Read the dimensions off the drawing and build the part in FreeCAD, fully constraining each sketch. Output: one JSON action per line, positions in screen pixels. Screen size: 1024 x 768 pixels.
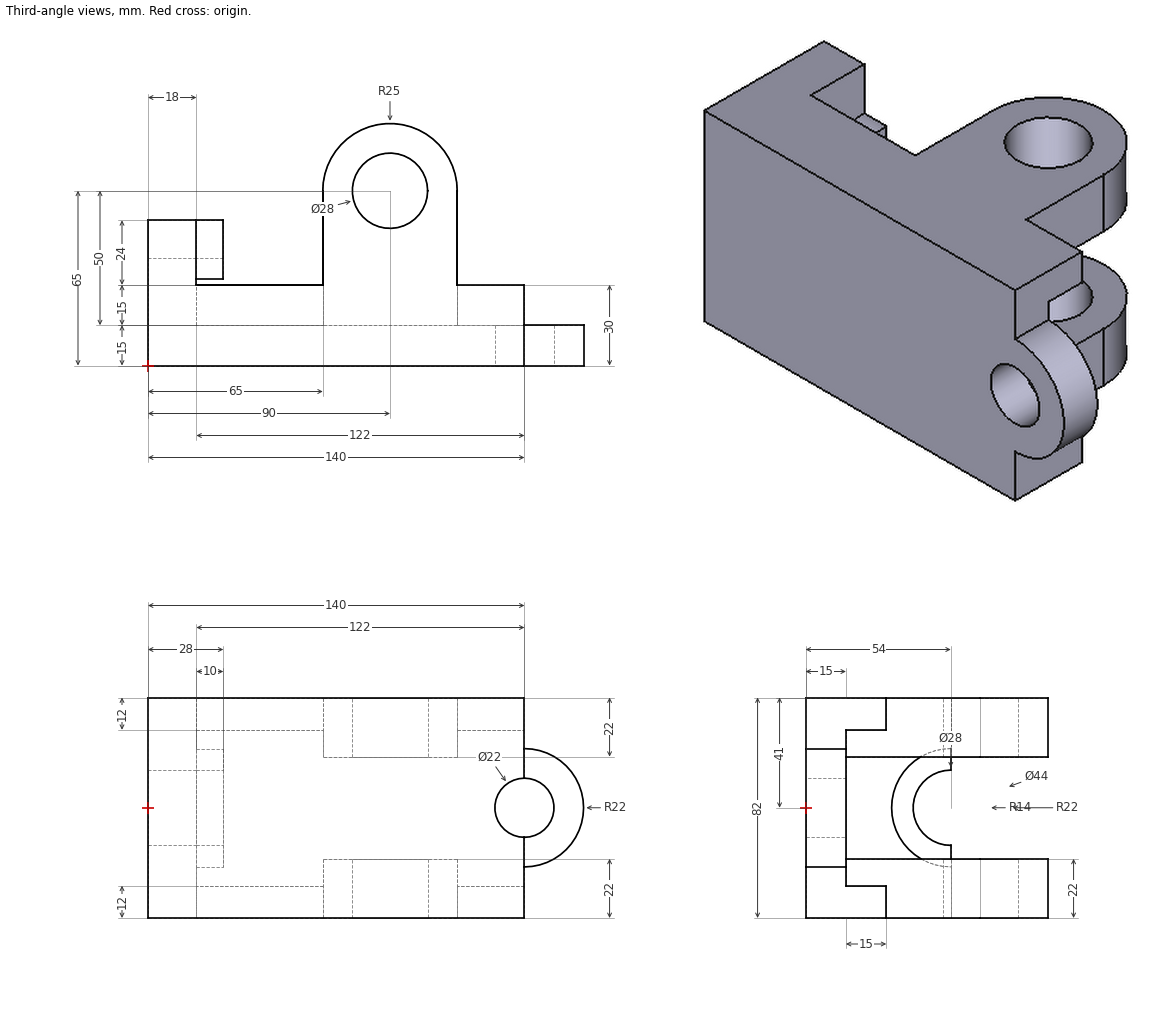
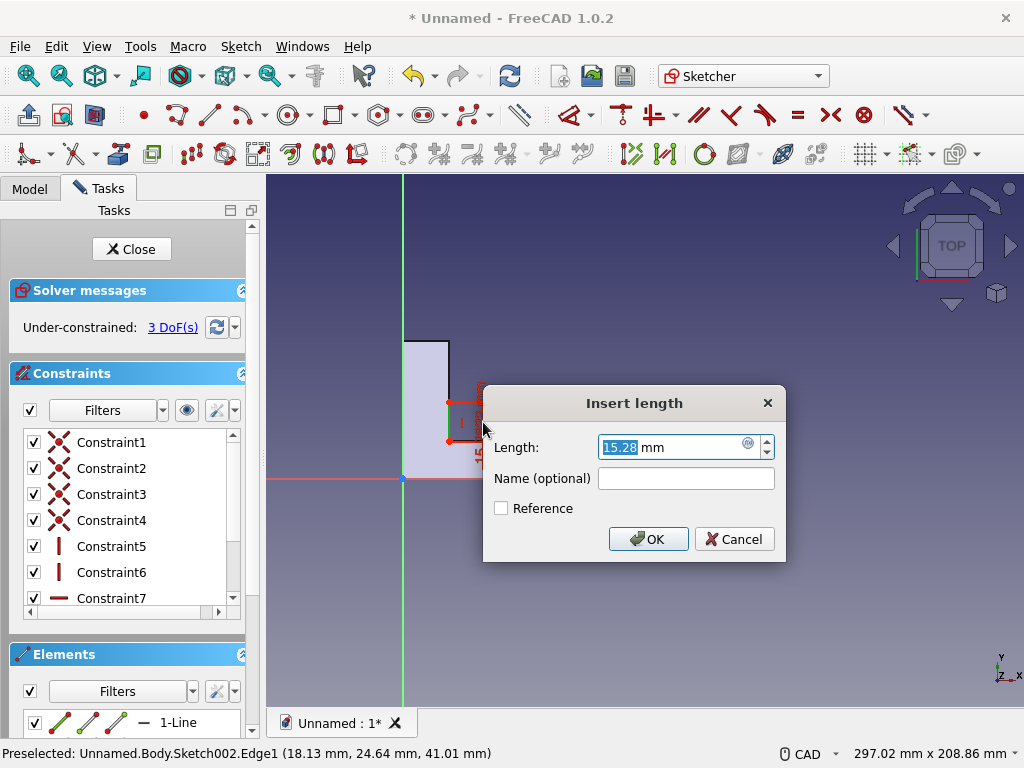
{"action": "type", "text": "15"}
{"action": "key", "text": "Return"}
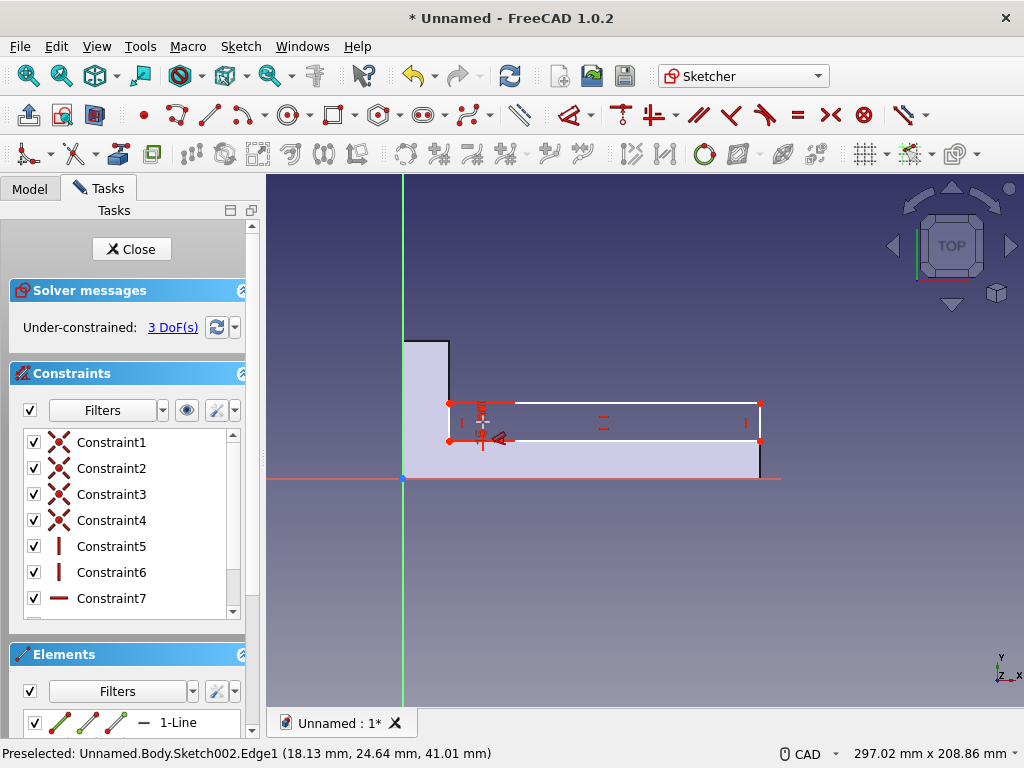
{"action": "left_click", "coordinate": [542, 441]}
{"action": "left_click", "coordinate": [605, 499]}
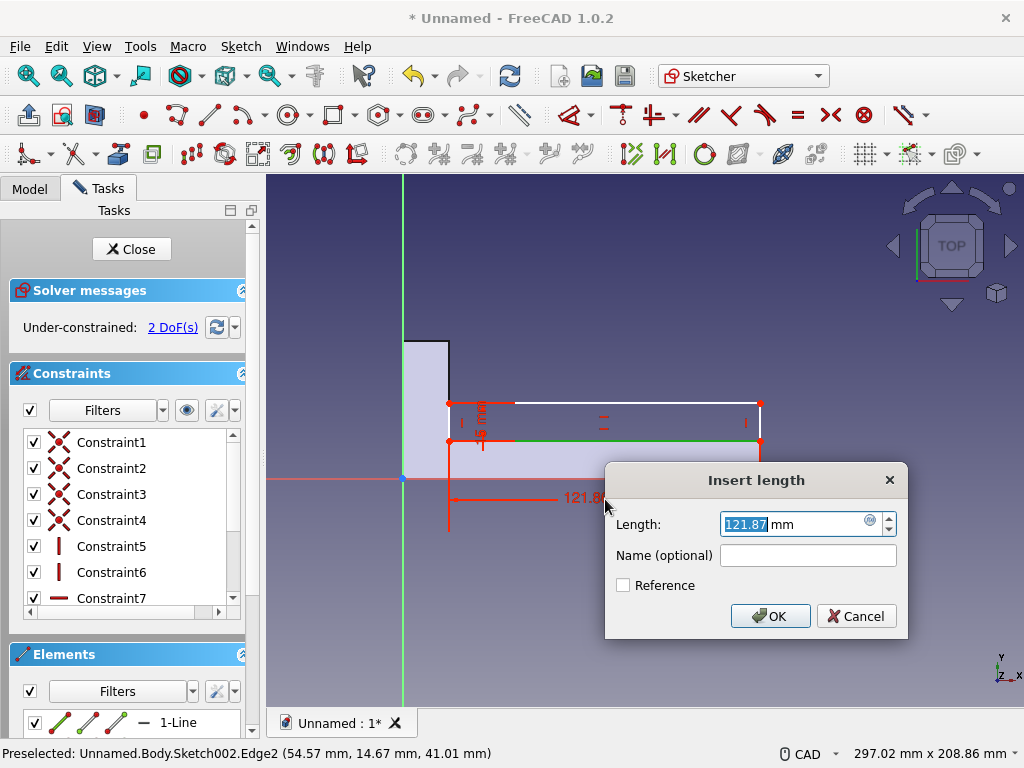
{"action": "type", "text": "122"}
{"action": "key", "text": "Return"}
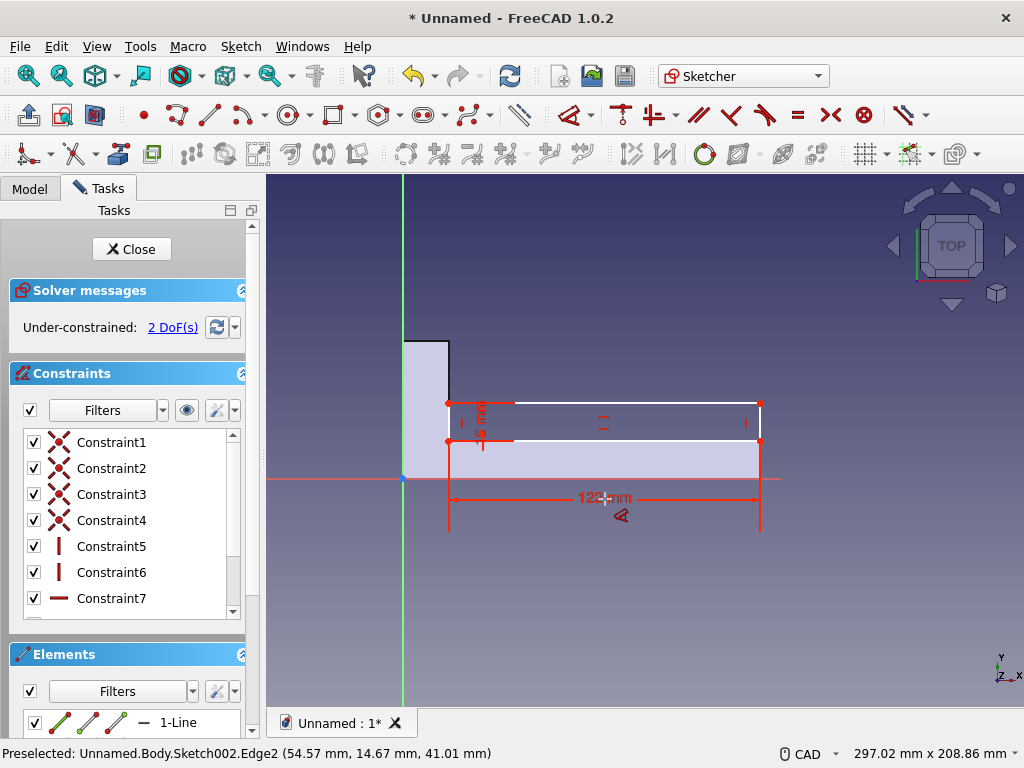
{"action": "left_click", "coordinate": [449, 403]}
{"action": "left_click", "coordinate": [426, 513]}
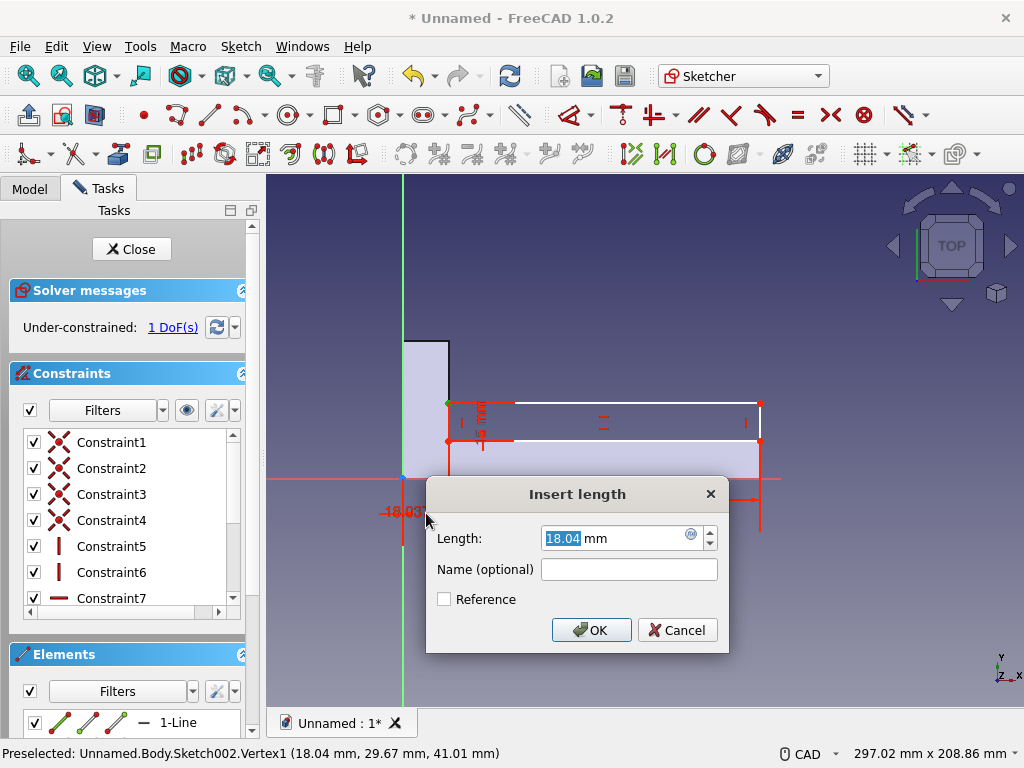
{"action": "type", "text": "18"}
{"action": "key", "text": "Return"}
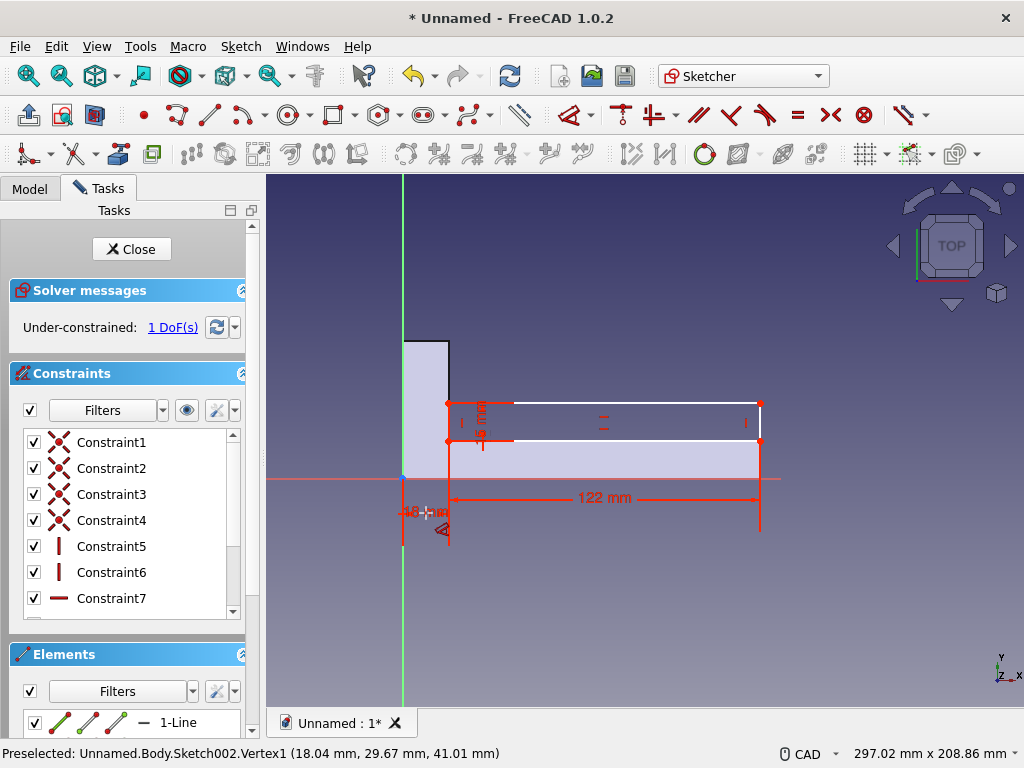
{"action": "left_click", "coordinate": [449, 403]}
{"action": "left_click", "coordinate": [369, 441]}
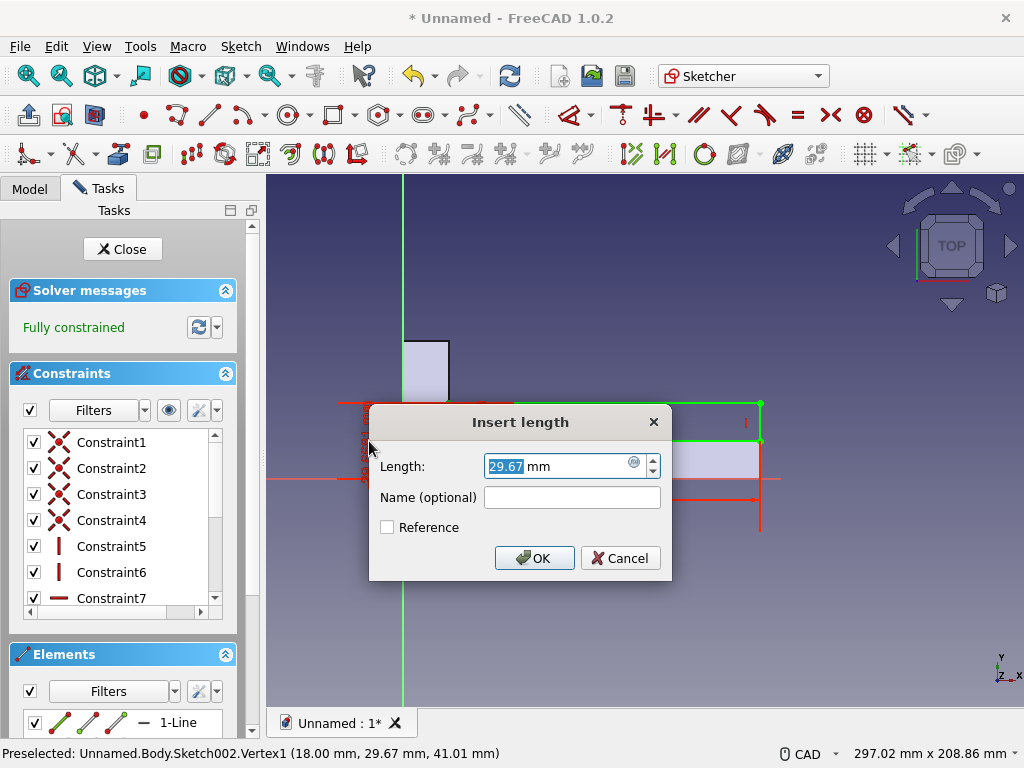
{"action": "type", "text": "30"}
{"action": "key", "text": "Return"}
{"action": "key", "text": "Escape"}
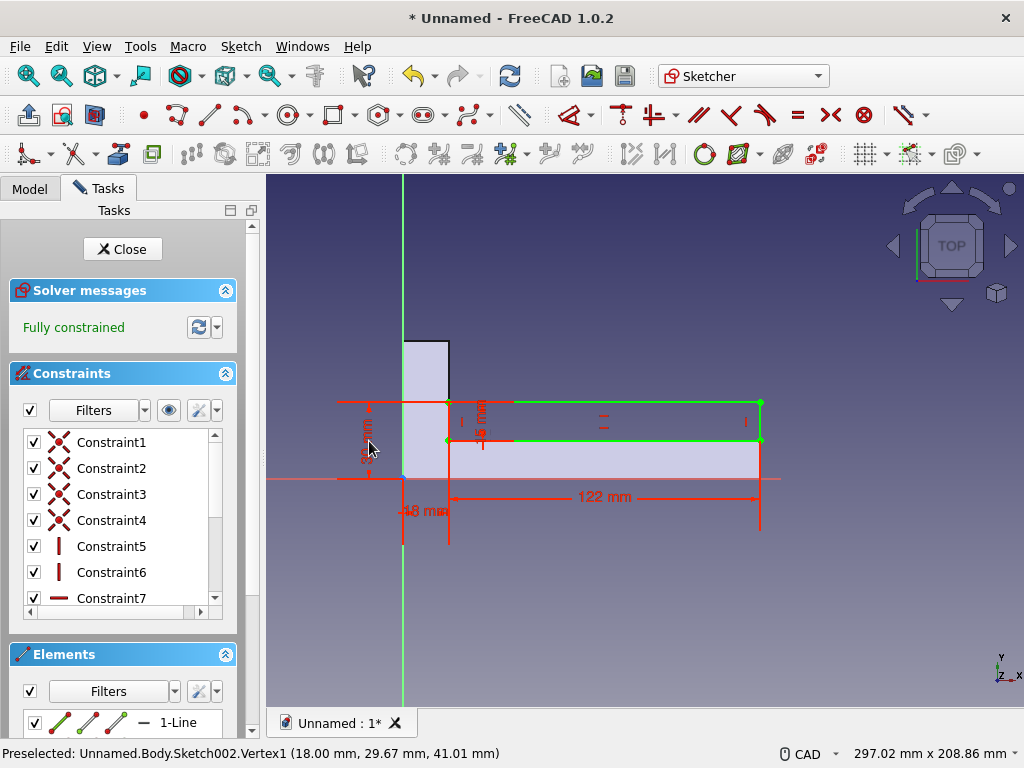
{"action": "left_click", "coordinate": [123, 249]}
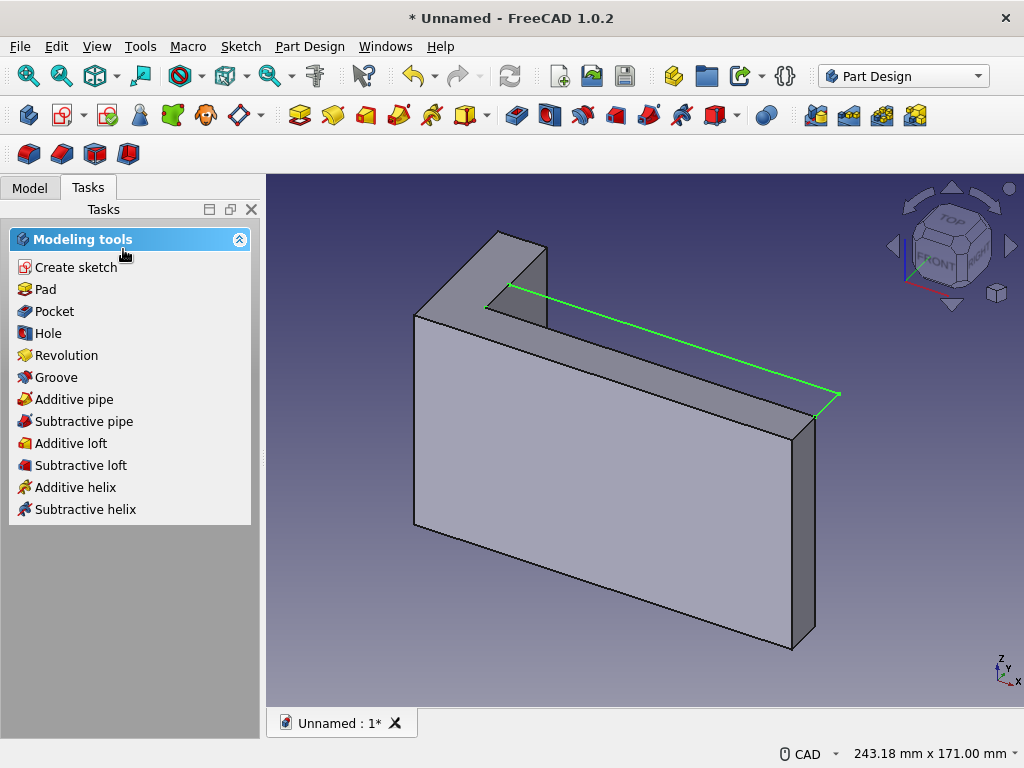
{"action": "left_click", "coordinate": [300, 116]}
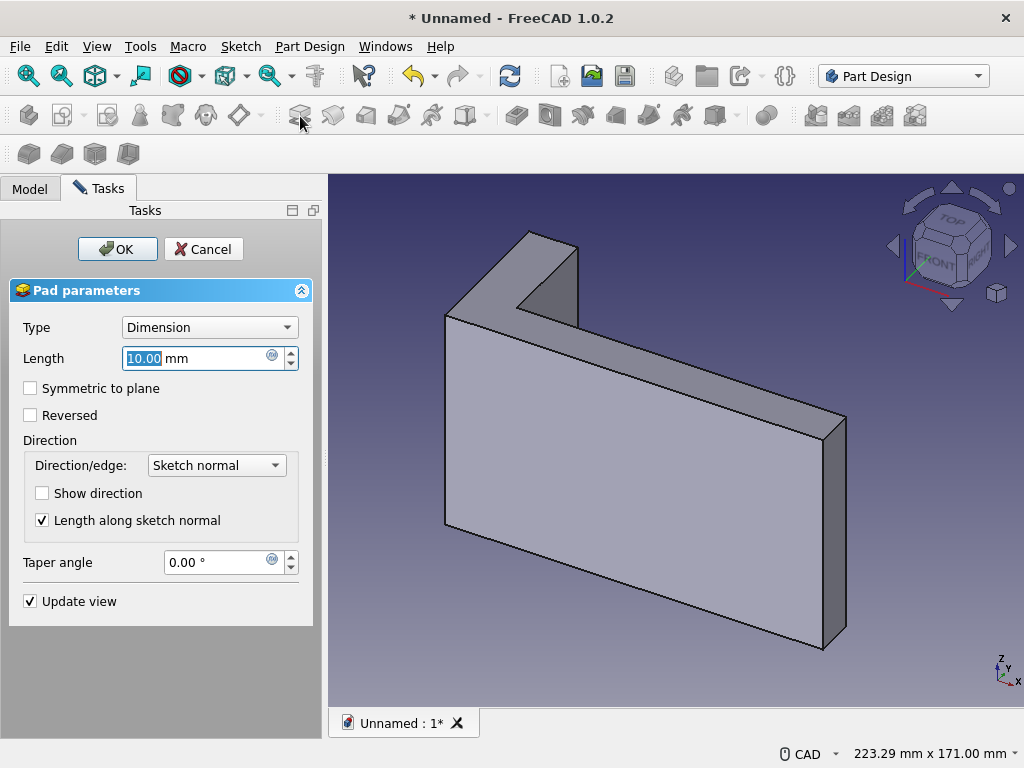
{"action": "type", "text": "12"}
{"action": "key", "text": "Tab"}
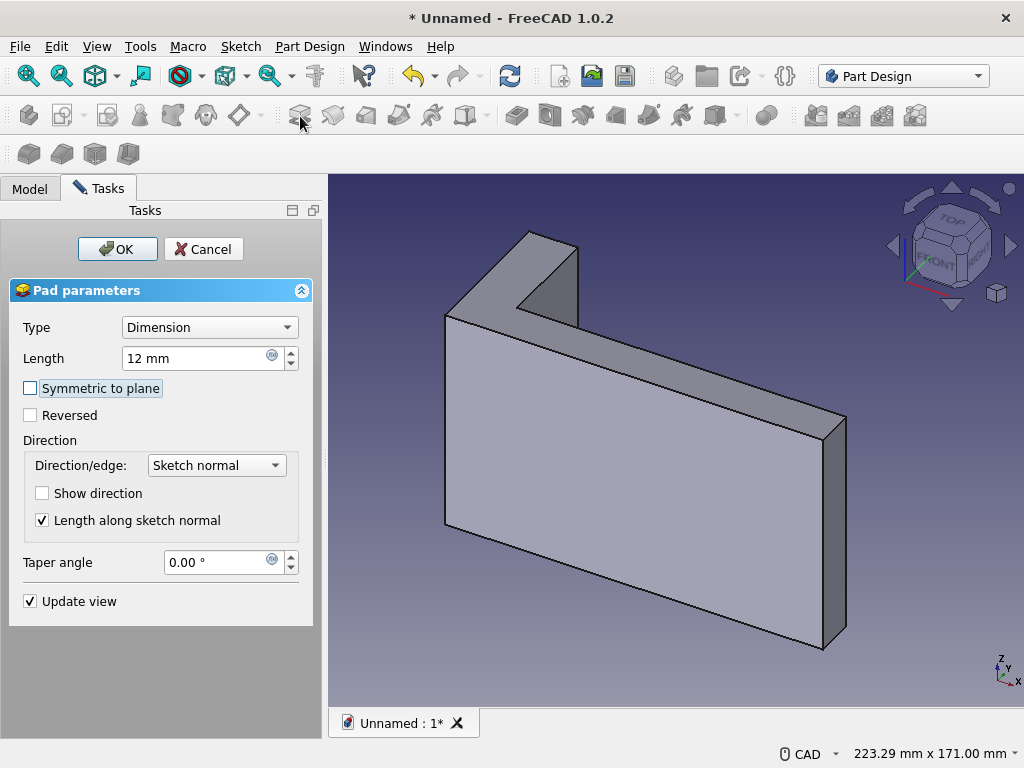
{"action": "left_click", "coordinate": [31, 415]}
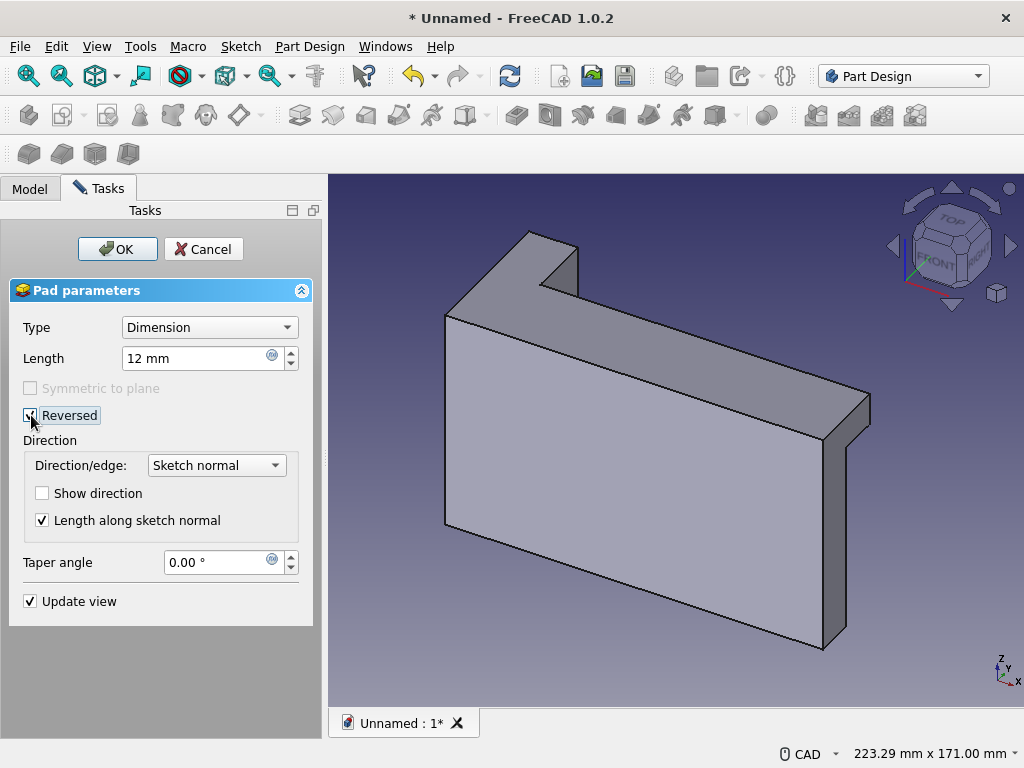
{"action": "left_click", "coordinate": [118, 249]}